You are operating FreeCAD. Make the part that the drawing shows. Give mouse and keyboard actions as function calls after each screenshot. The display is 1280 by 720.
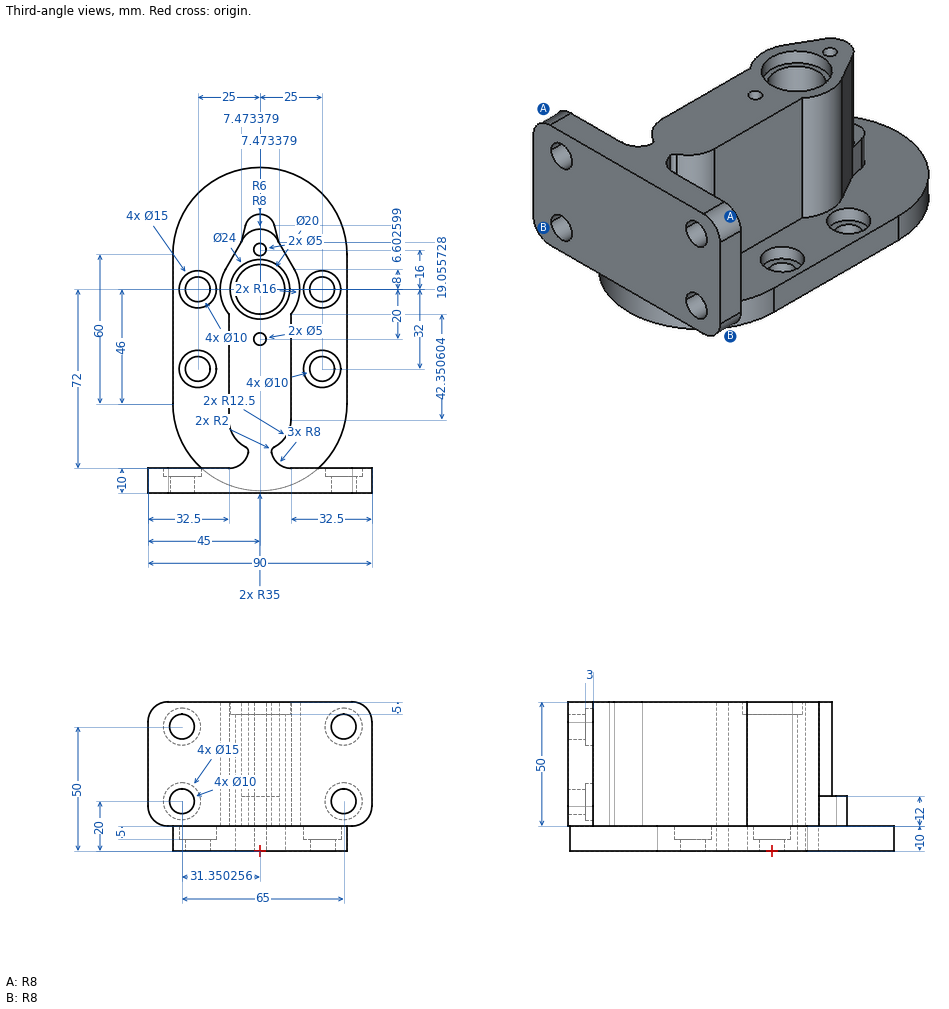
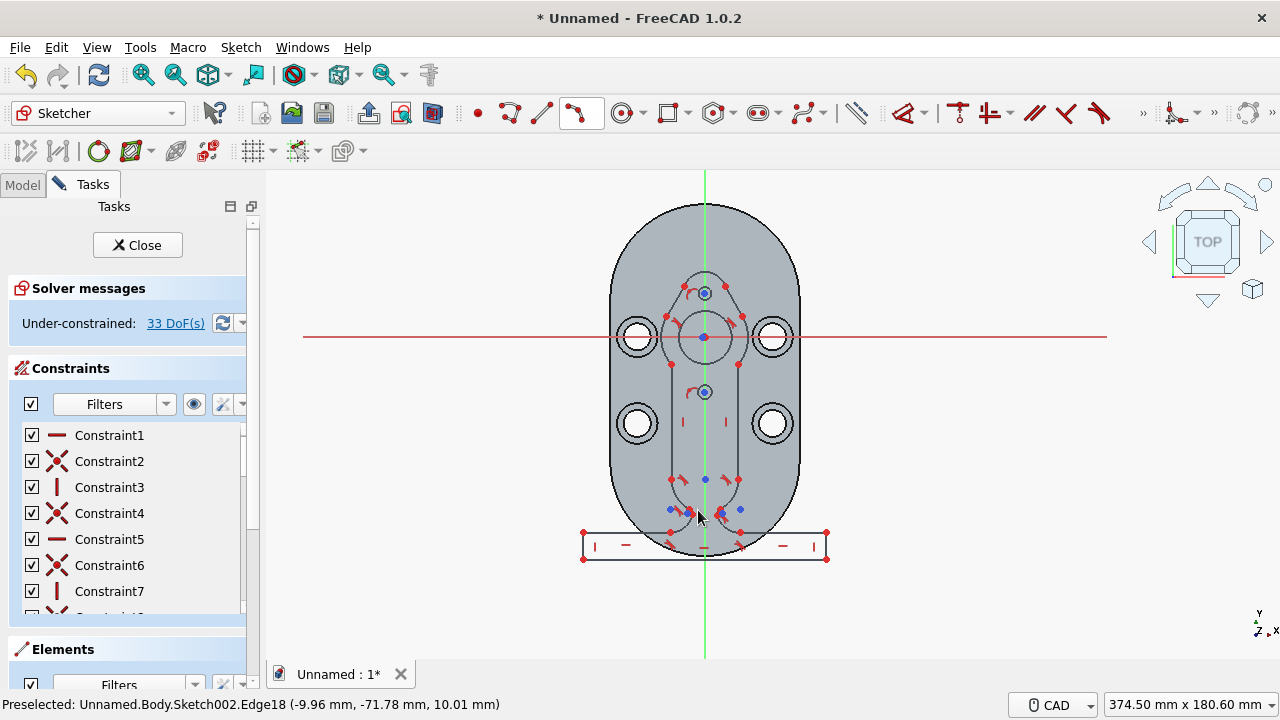
click(724, 319)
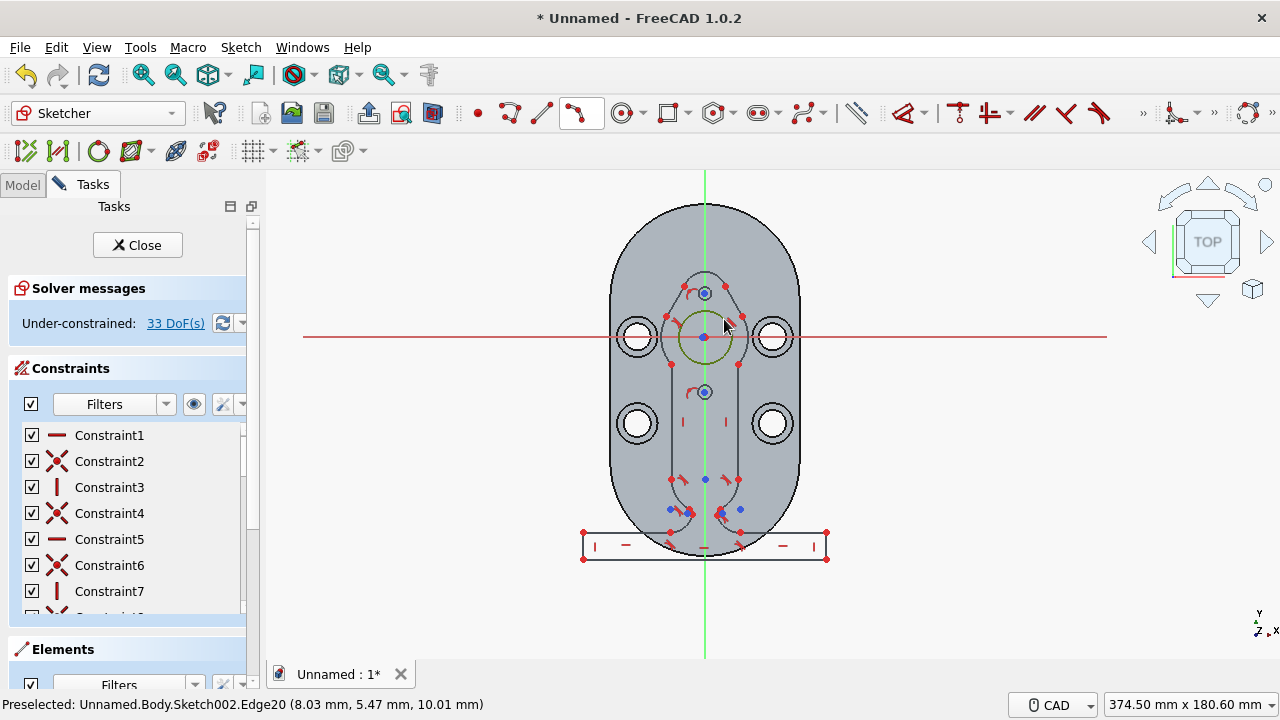
click(664, 351)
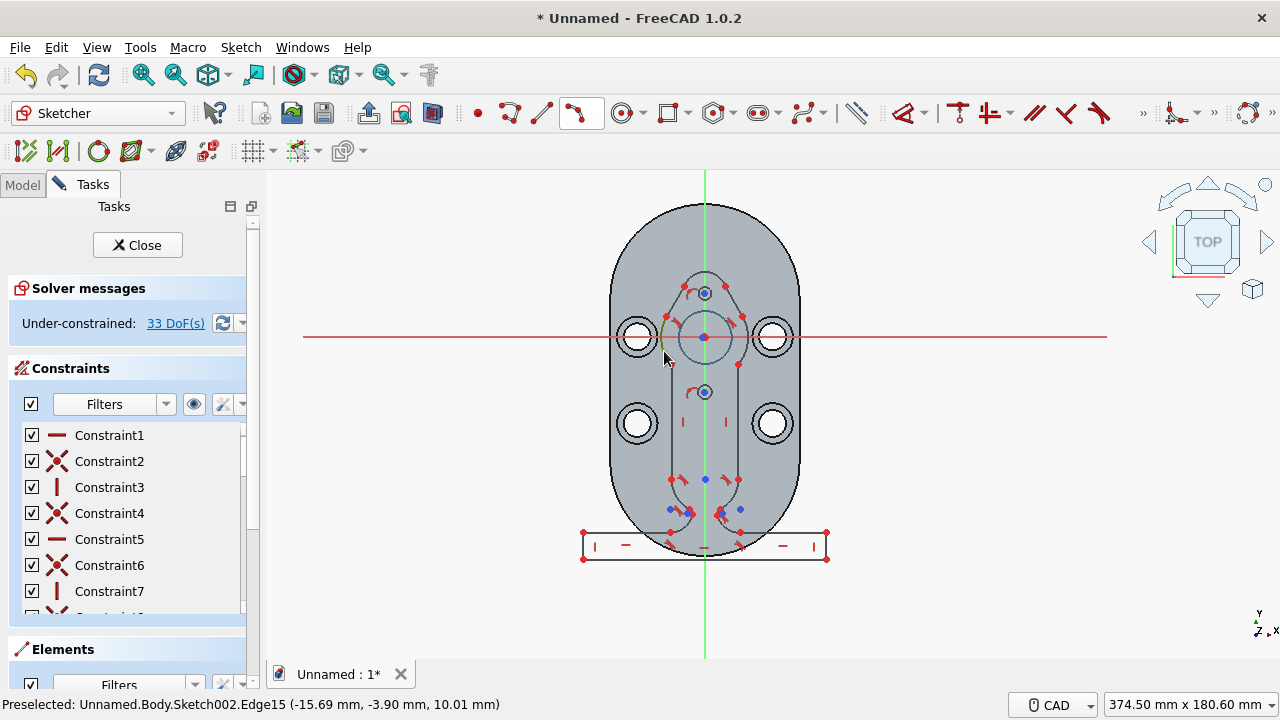
click(958, 114)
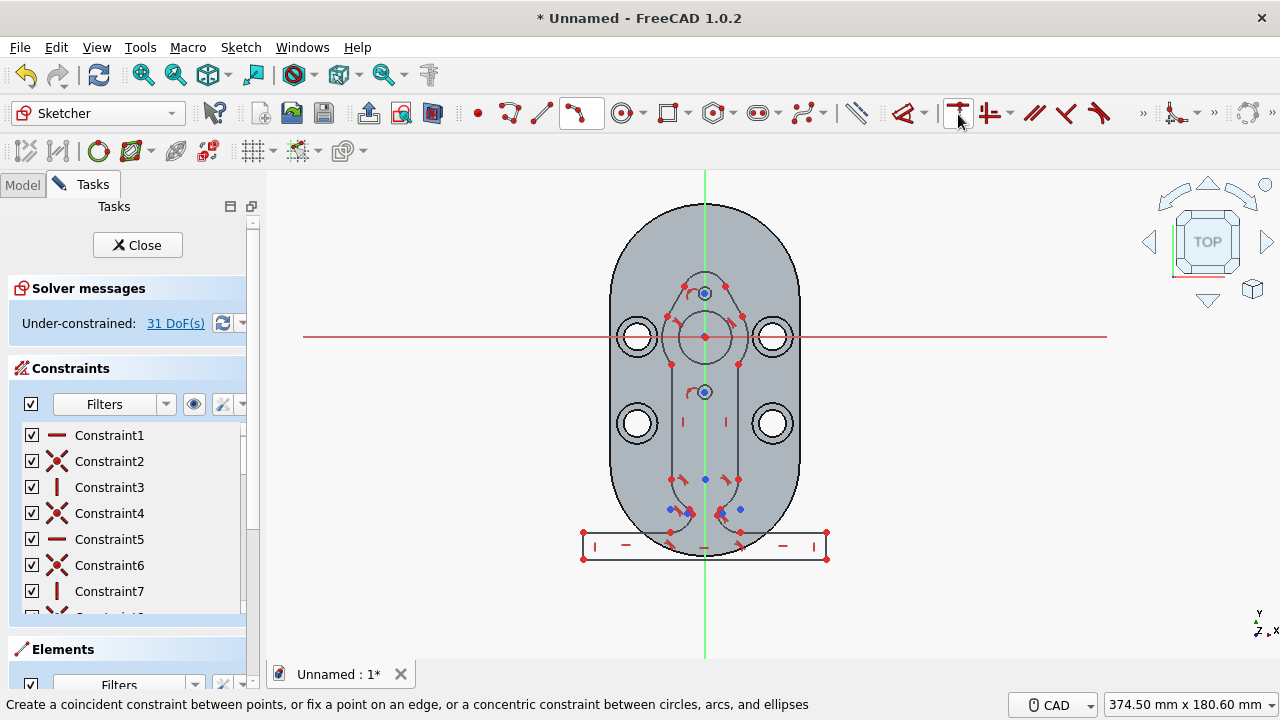
scroll(729, 503, up, 2)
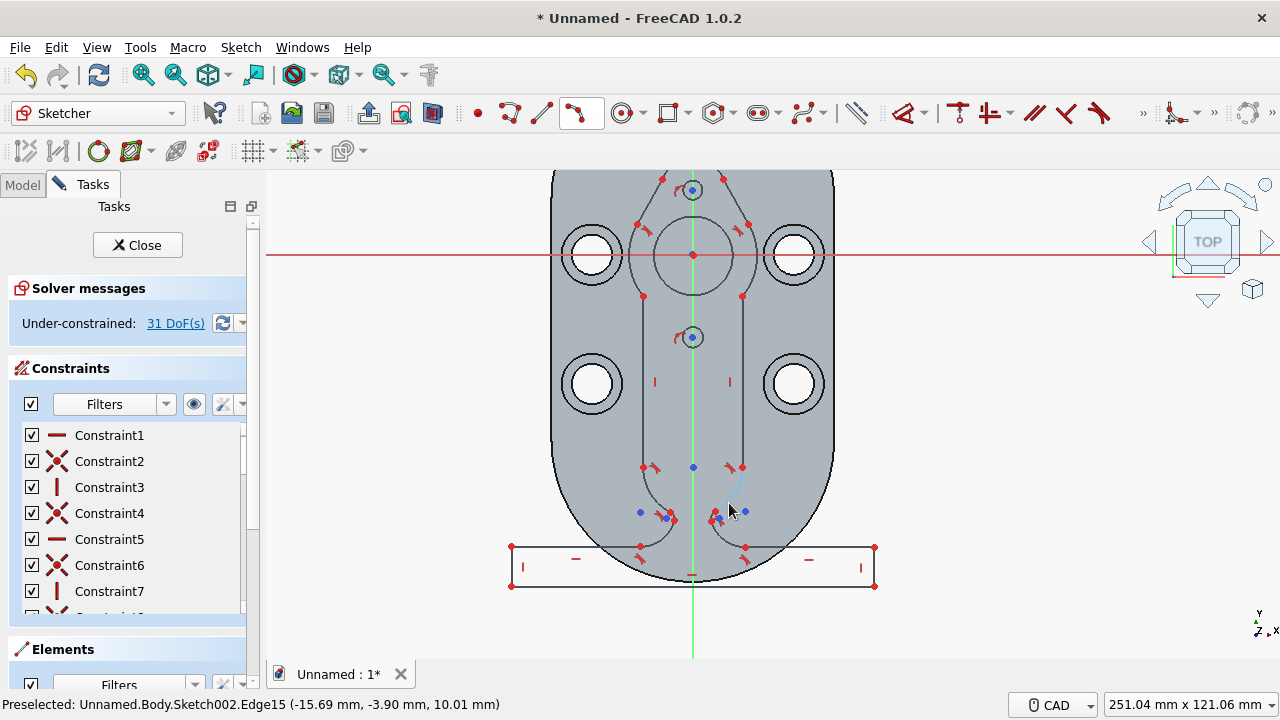
click(729, 502)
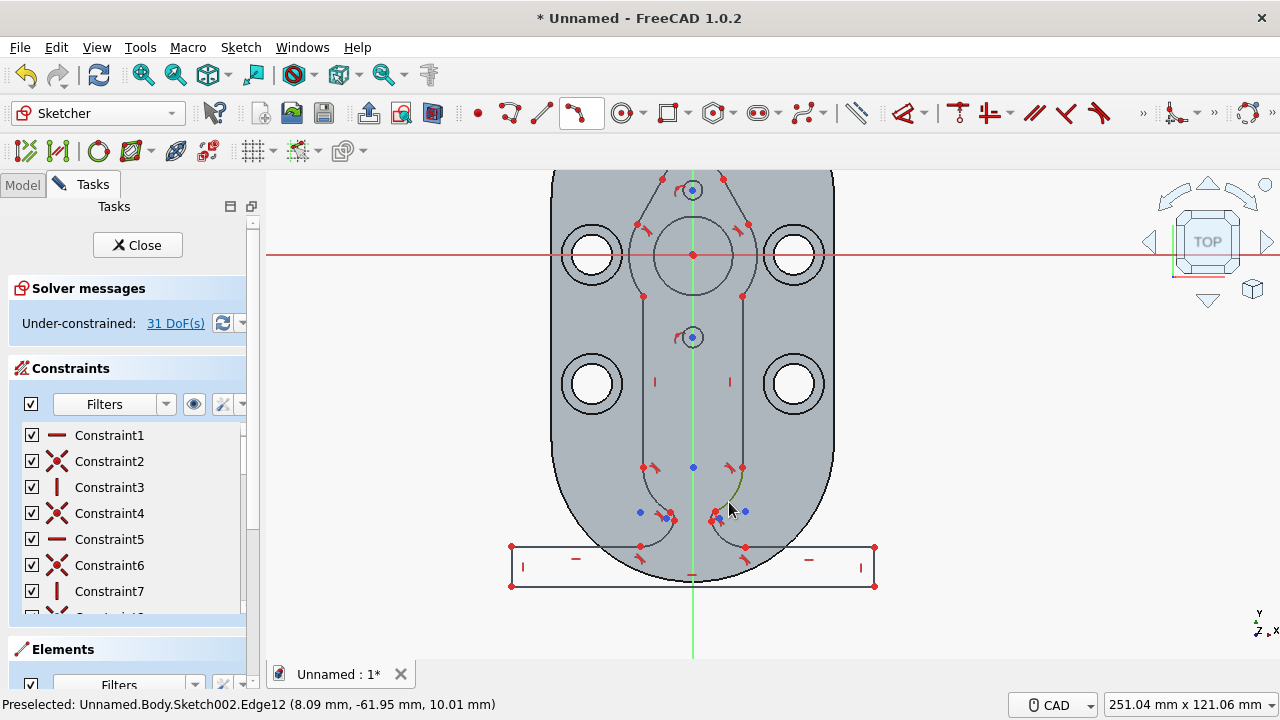
click(646, 484)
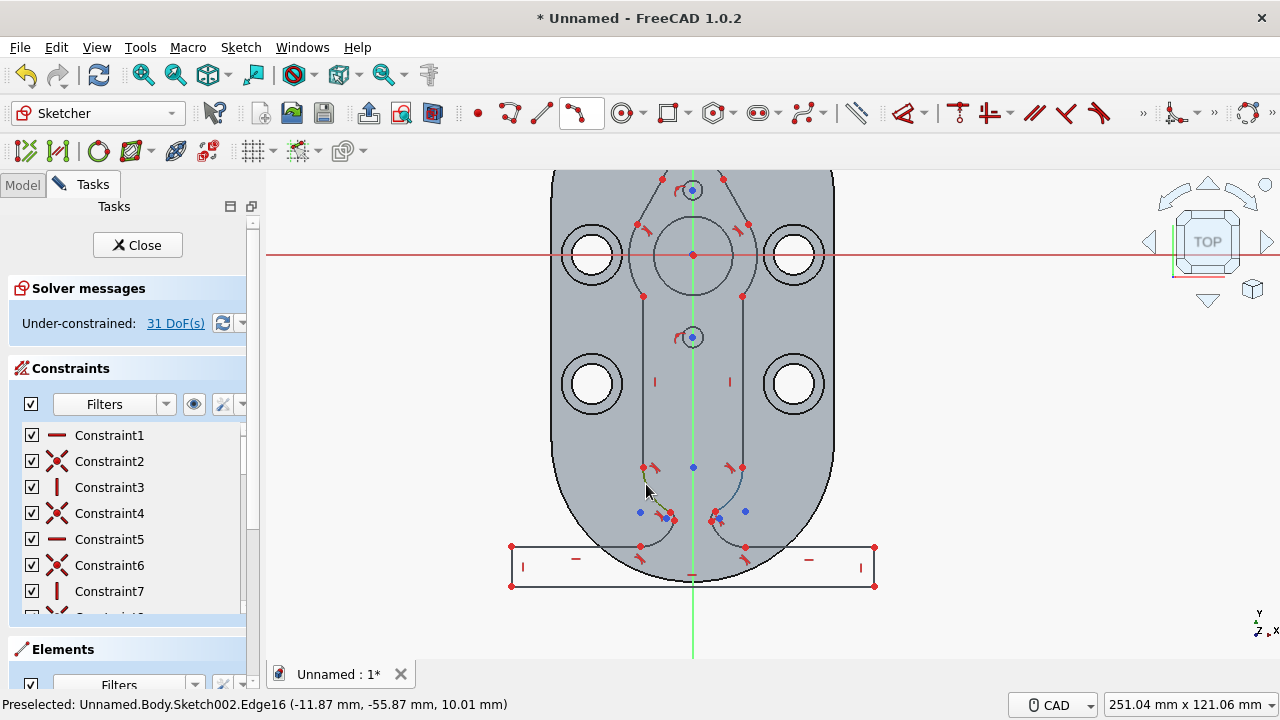
click(958, 114)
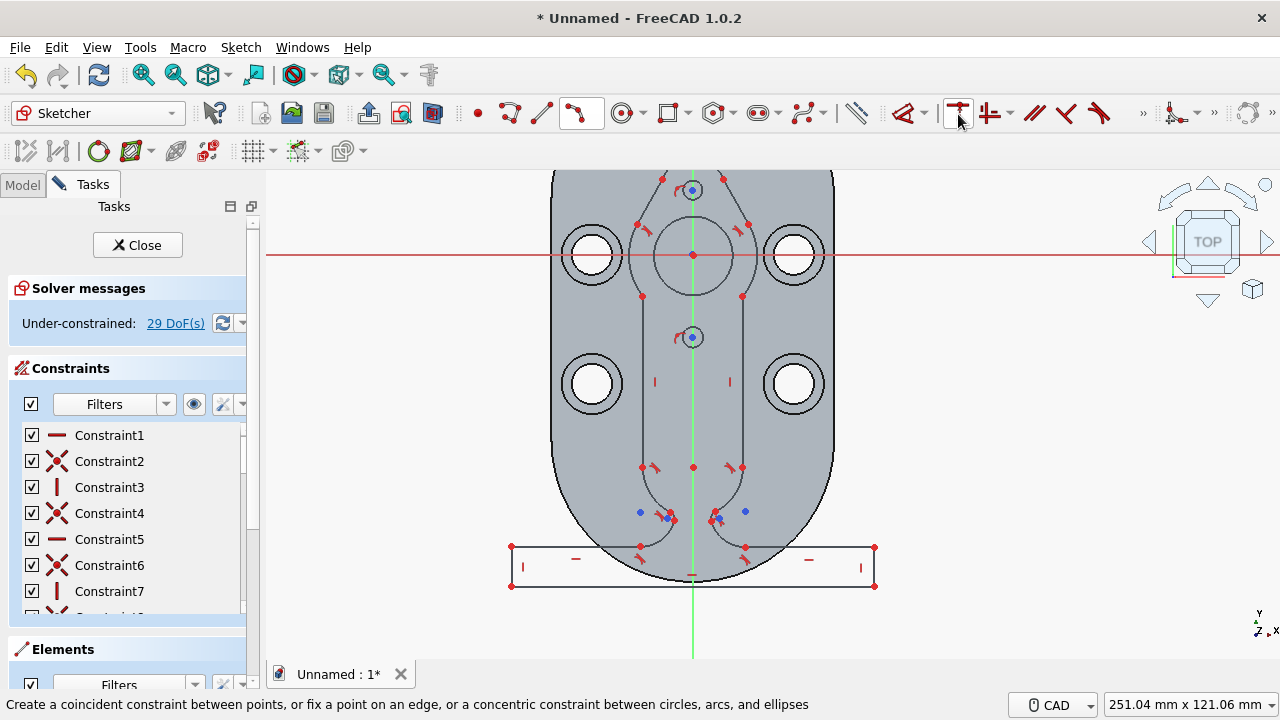
scroll(693, 255, up, 9)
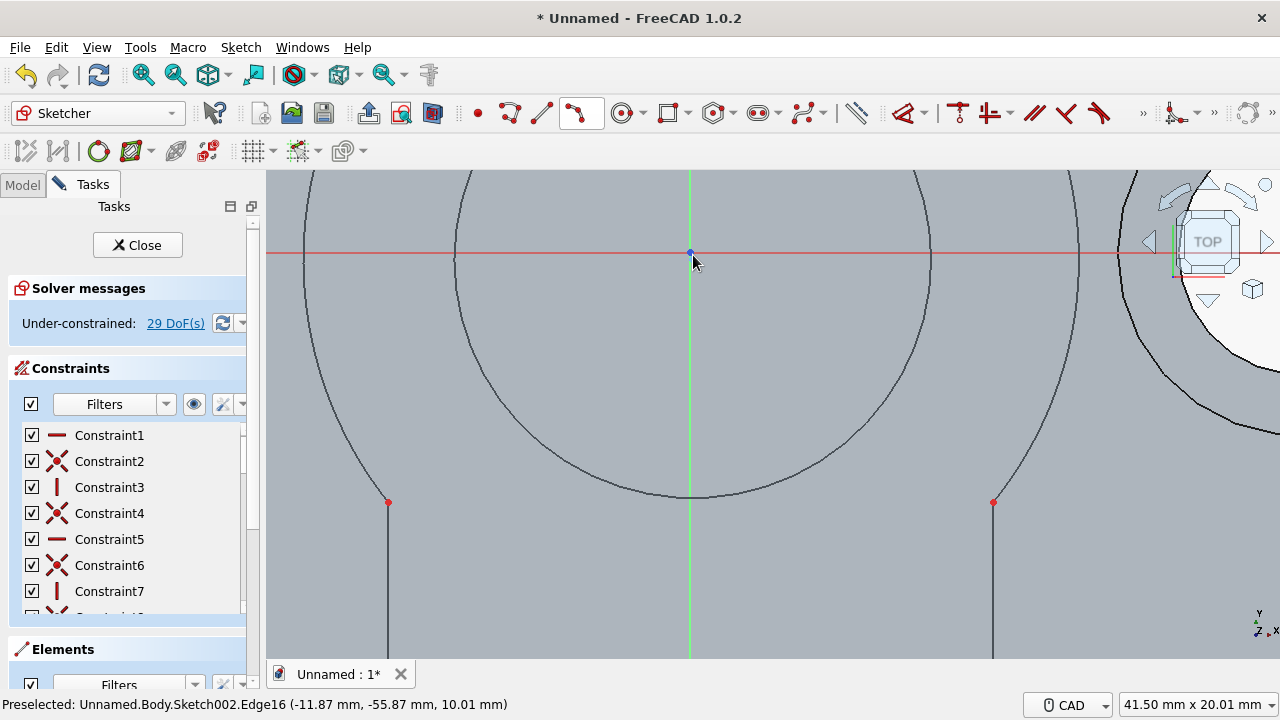
drag(680, 243, 703, 270)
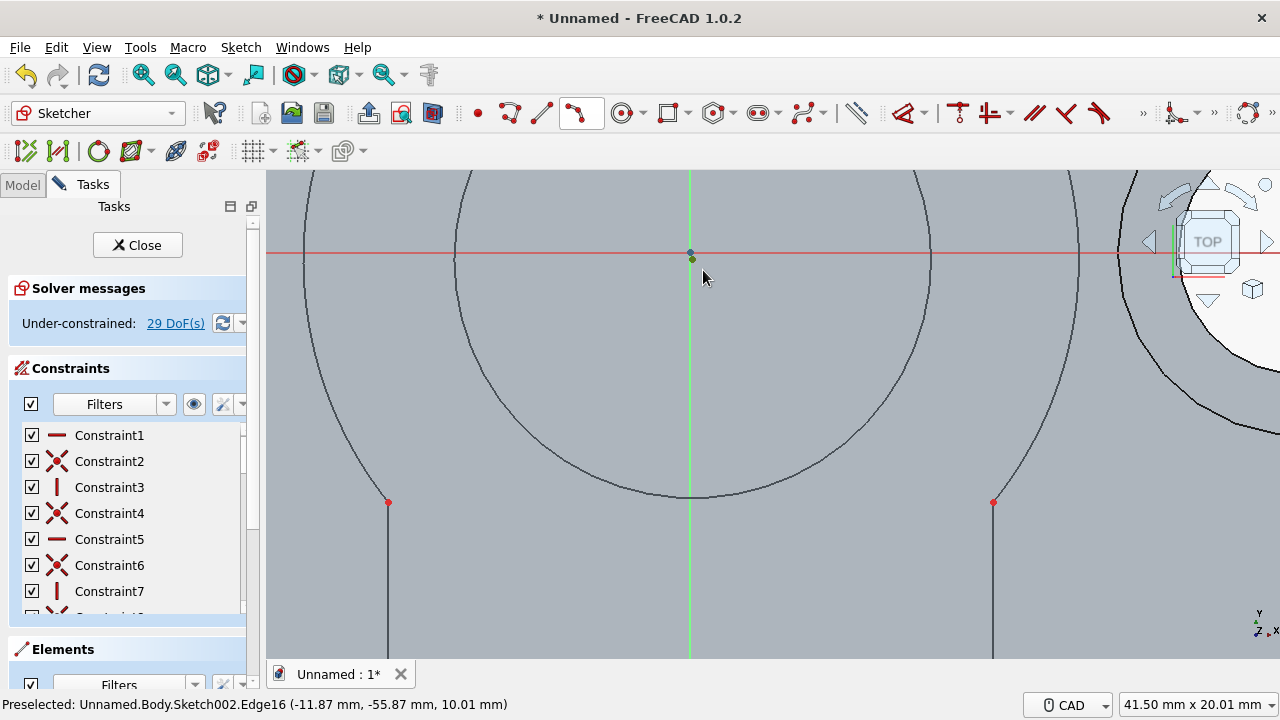
click(958, 114)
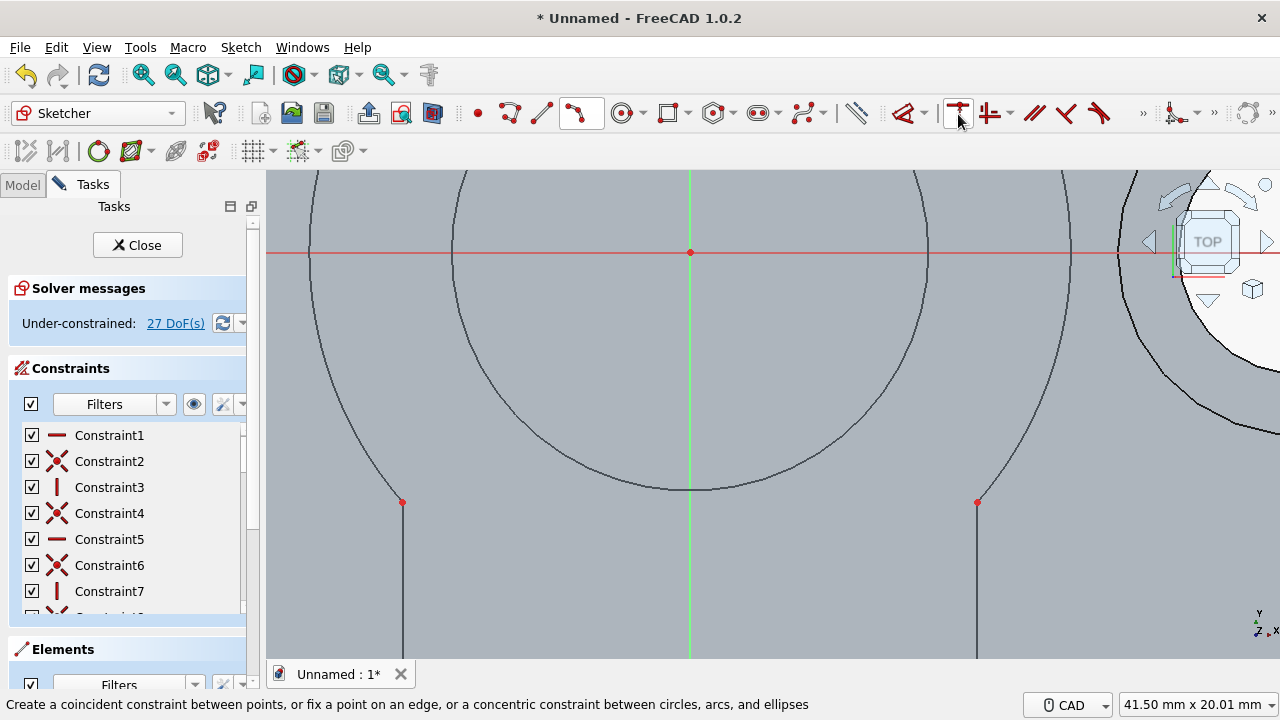
scroll(706, 347, down, 11)